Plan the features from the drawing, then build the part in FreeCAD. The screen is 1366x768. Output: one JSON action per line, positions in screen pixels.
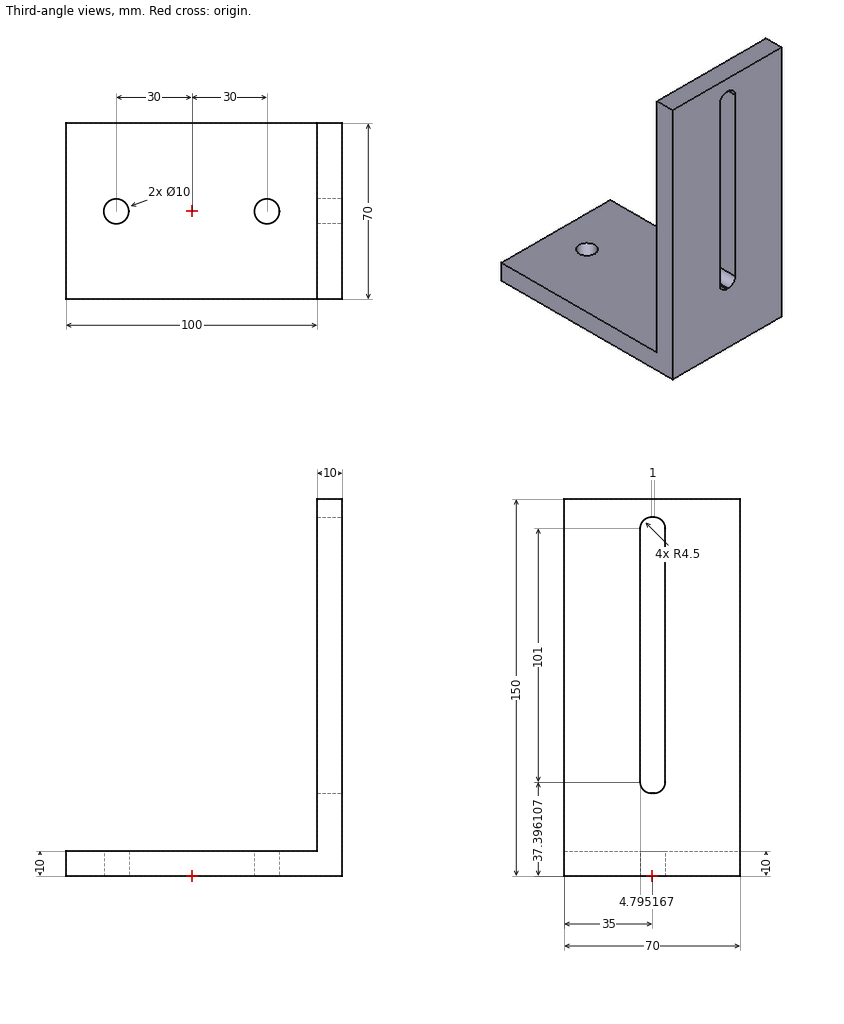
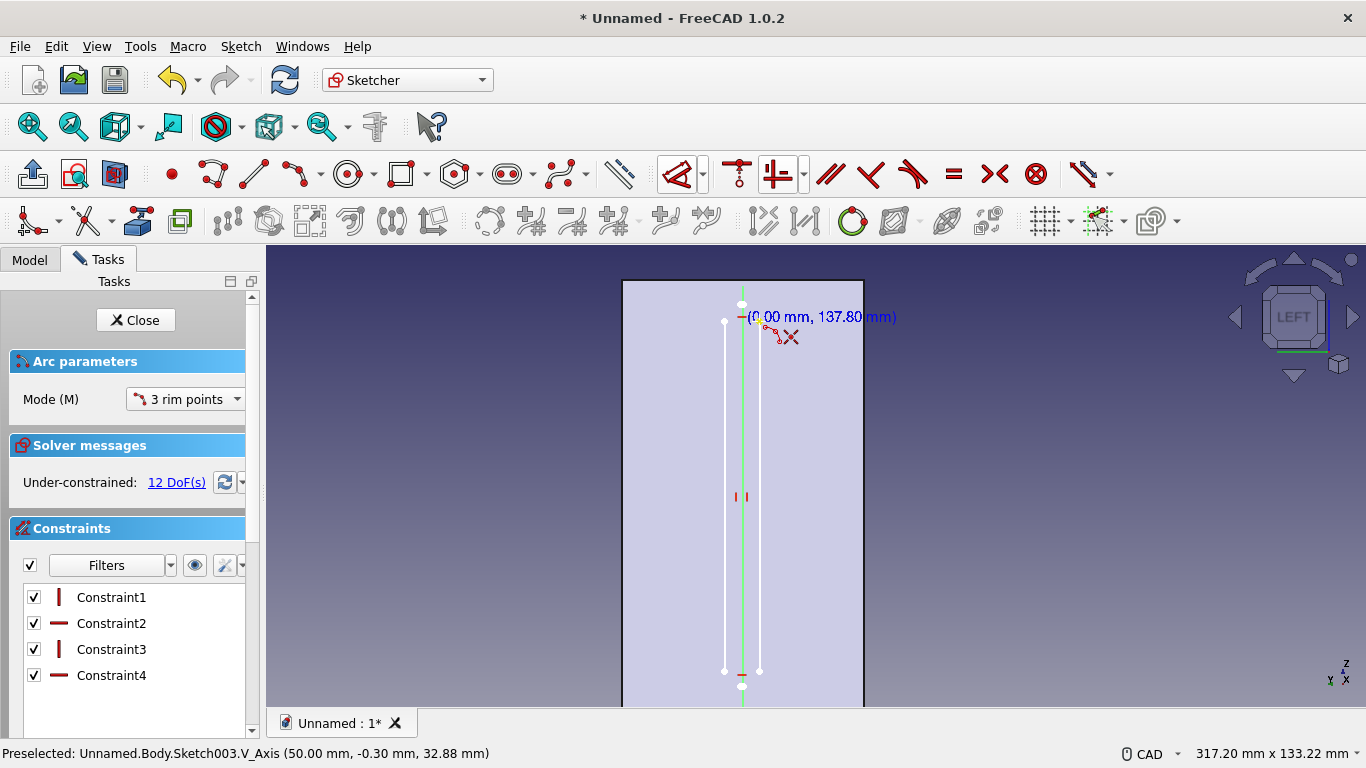
{"action": "left_click", "coordinate": [760, 321]}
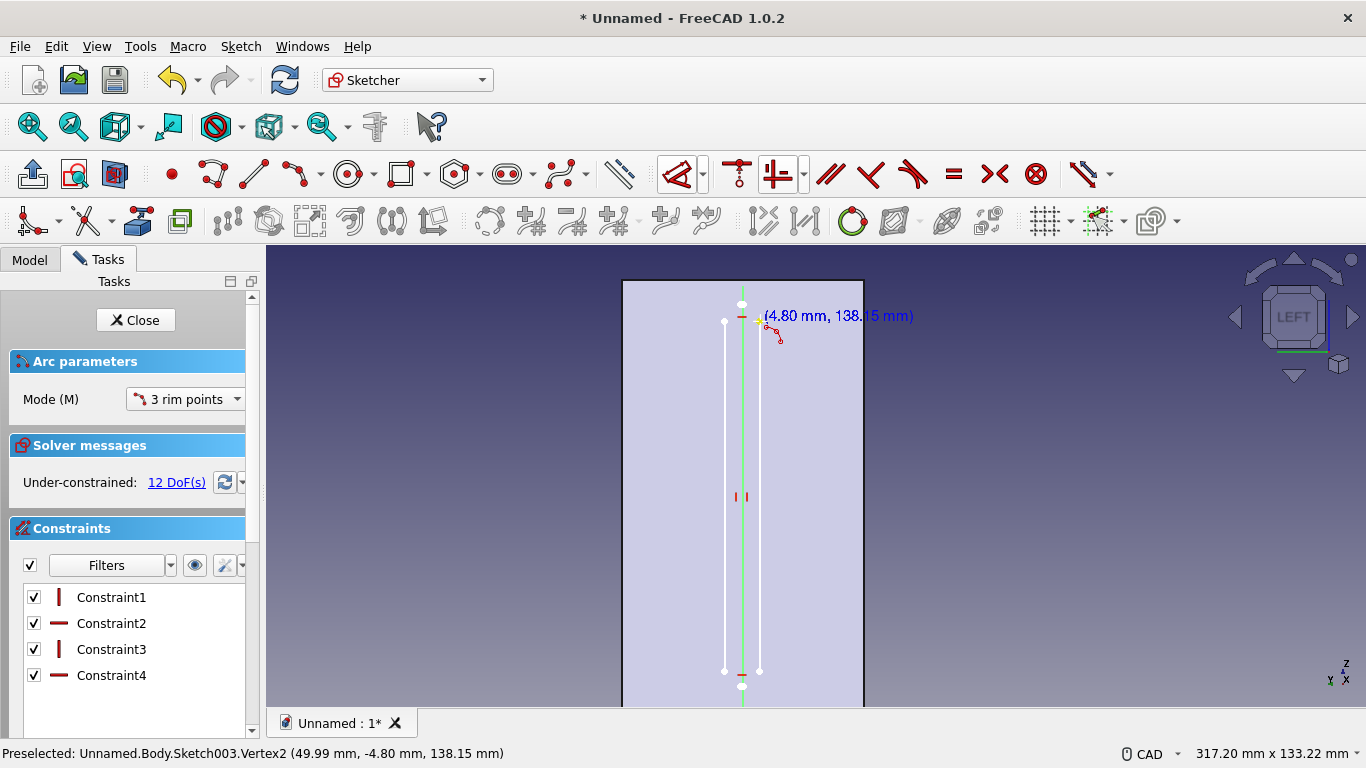
{"action": "scroll", "coordinate": [744, 305], "scroll_direction": "up", "scroll_amount": 14}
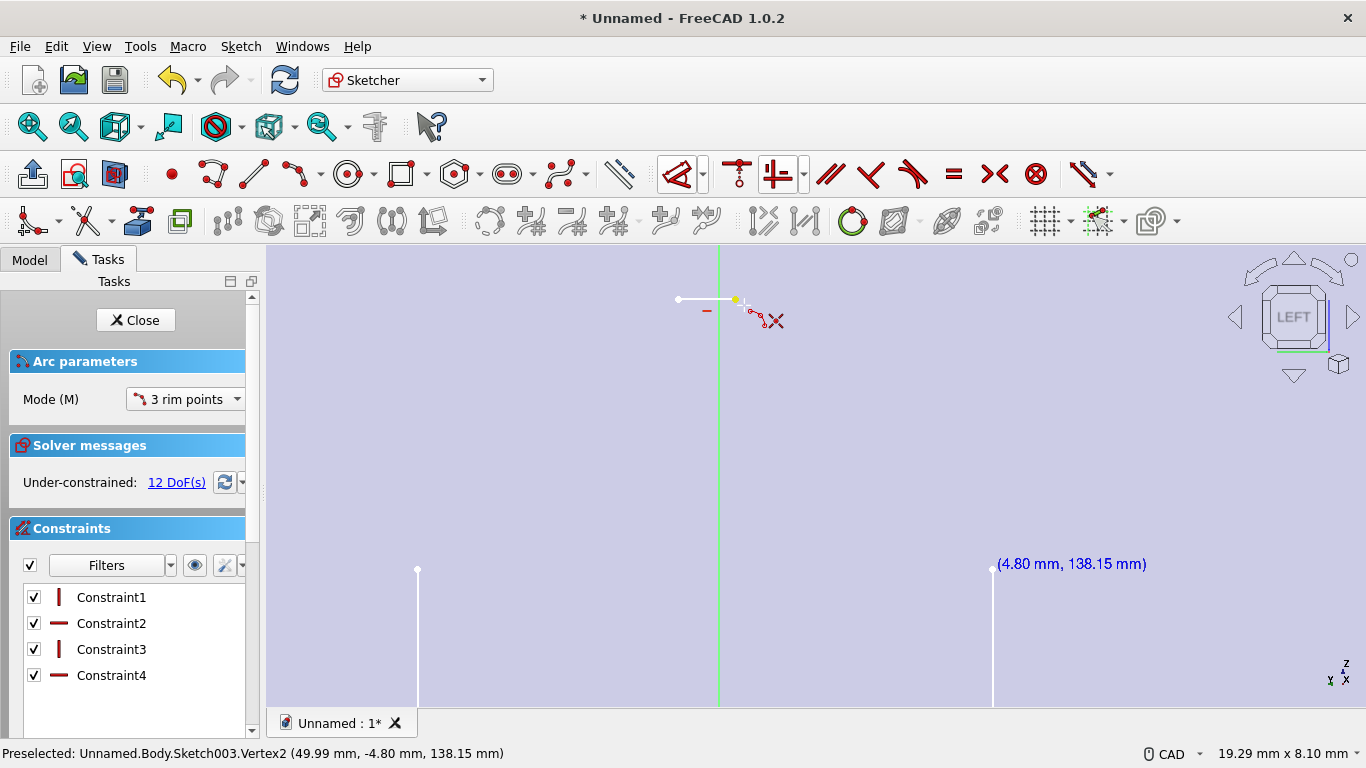
{"action": "left_click", "coordinate": [736, 299]}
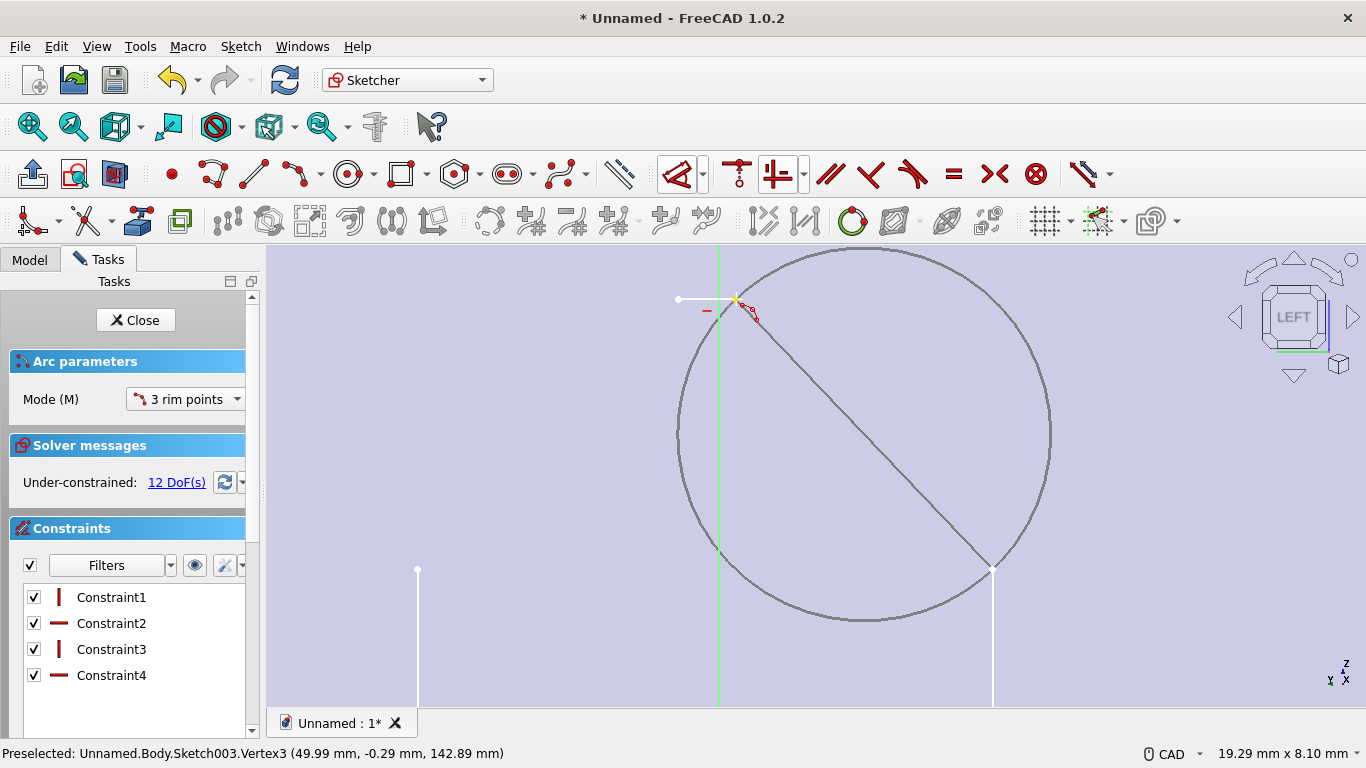
{"action": "scroll", "coordinate": [749, 310], "scroll_direction": "down", "scroll_amount": 16}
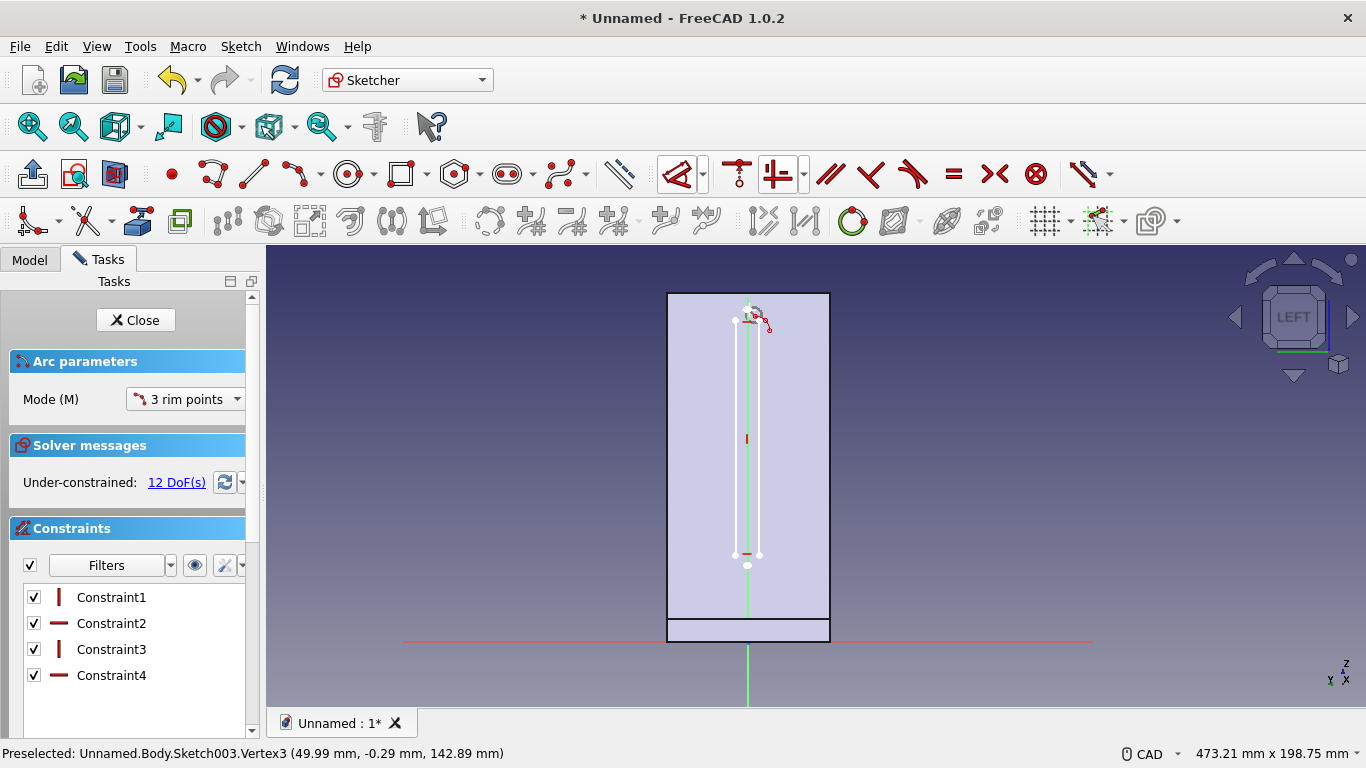
{"action": "scroll", "coordinate": [756, 313], "scroll_direction": "up", "scroll_amount": 9}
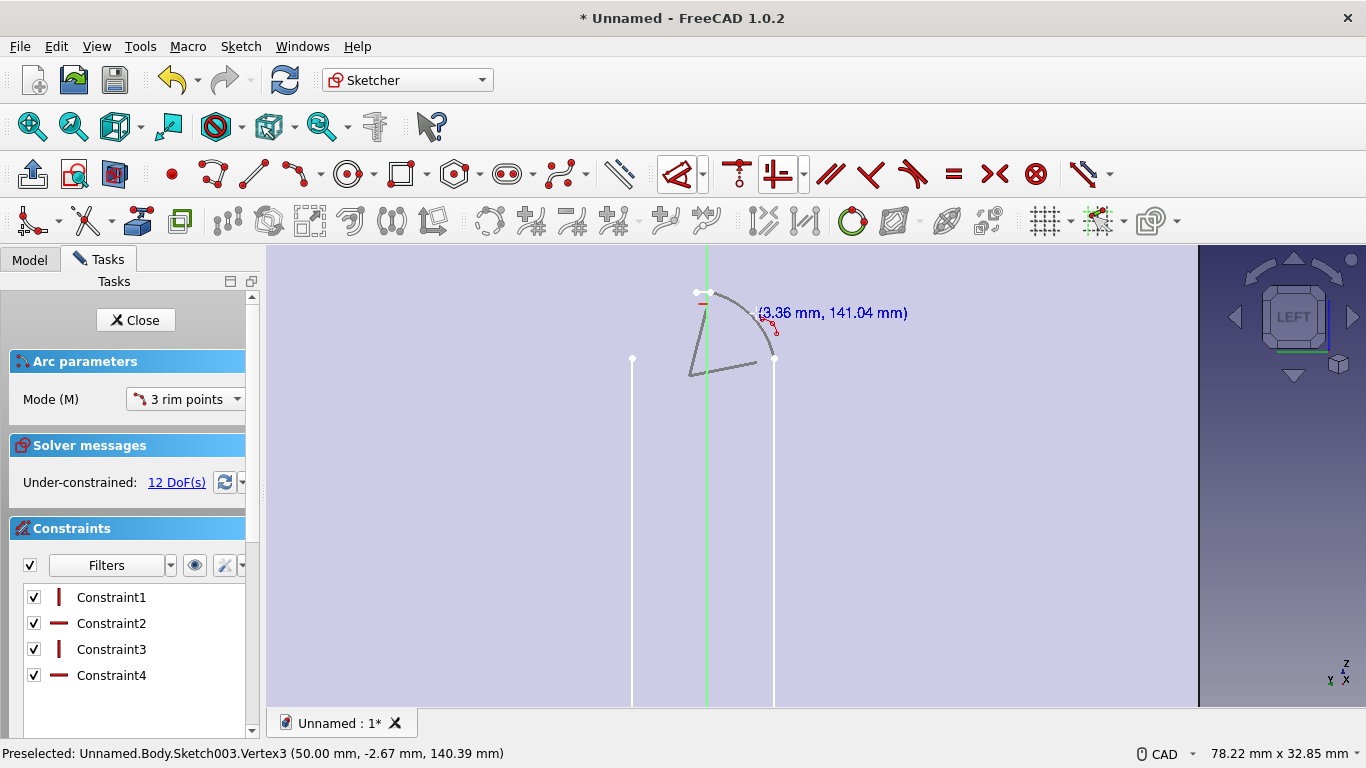
{"action": "left_click", "coordinate": [755, 311]}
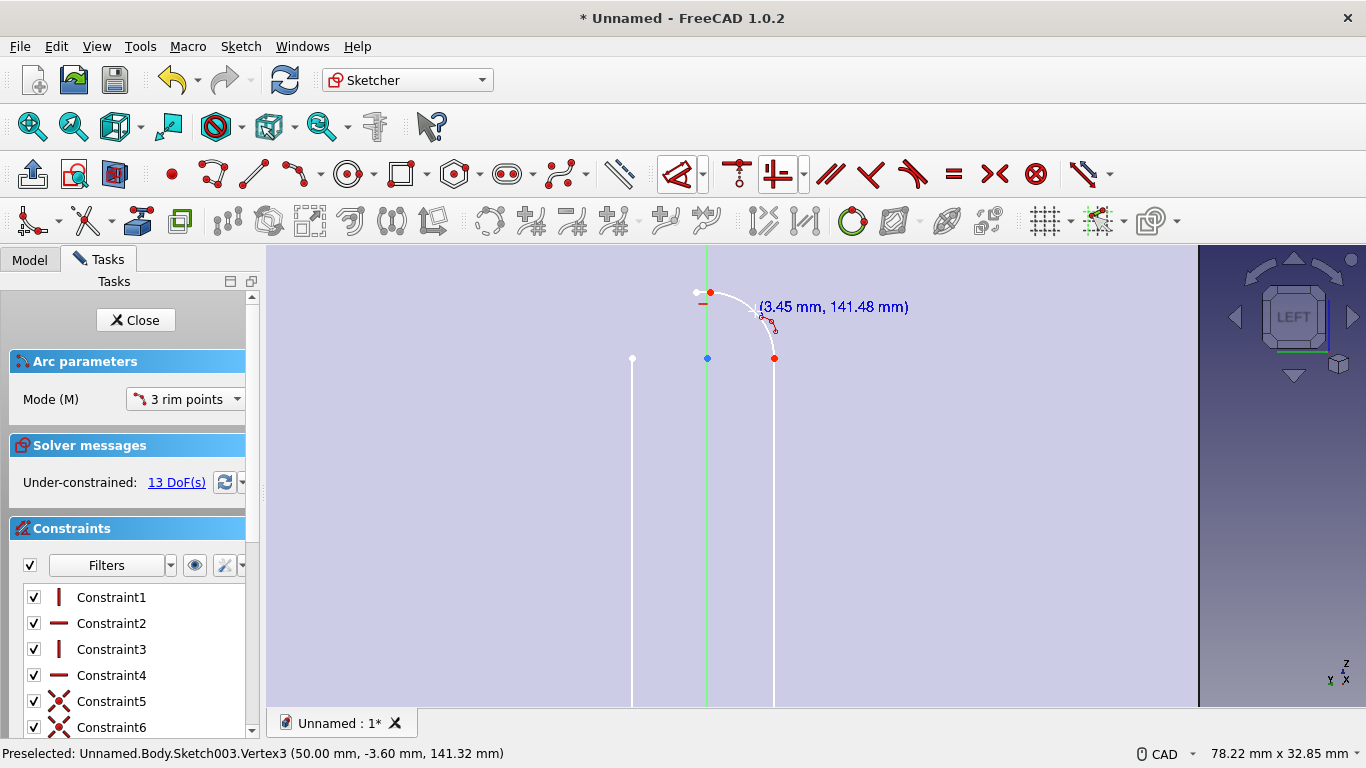
{"action": "scroll", "coordinate": [697, 292], "scroll_direction": "up", "scroll_amount": 5}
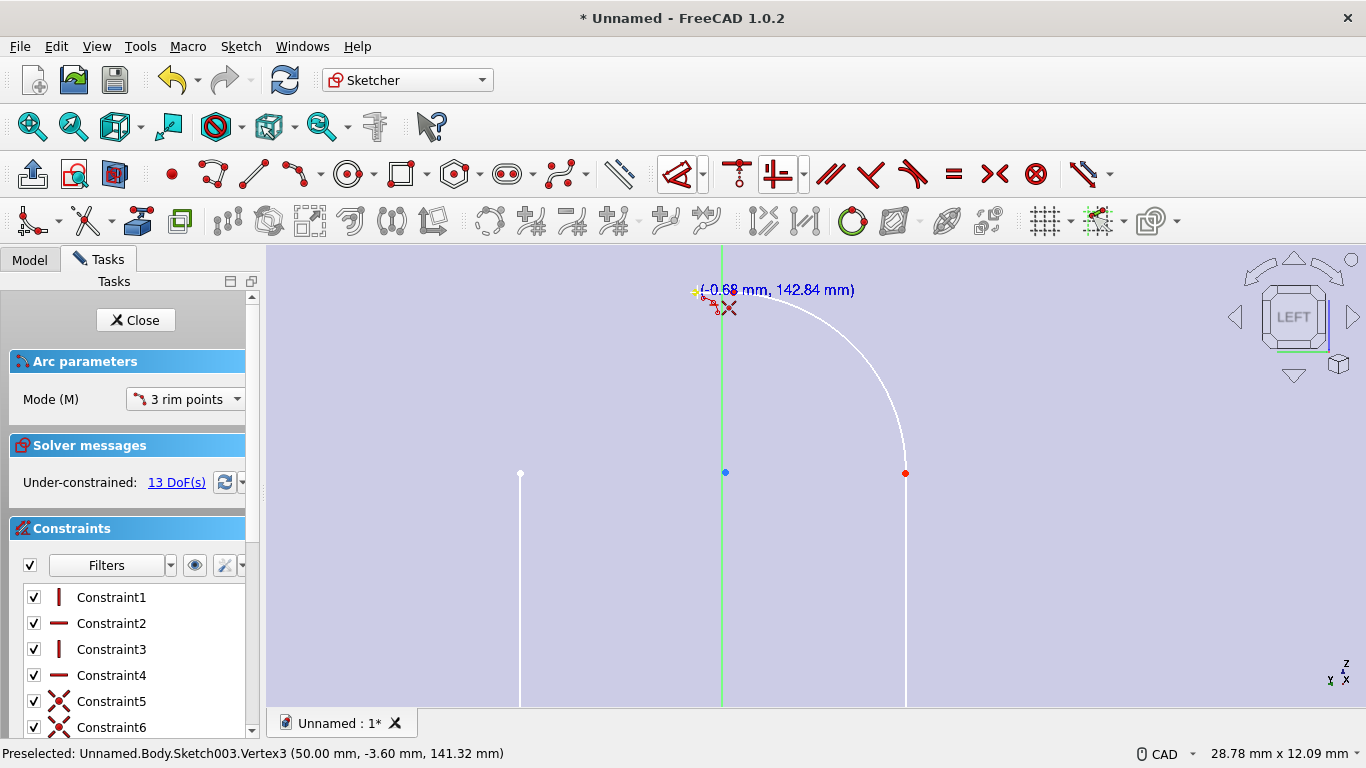
{"action": "left_click", "coordinate": [695, 293]}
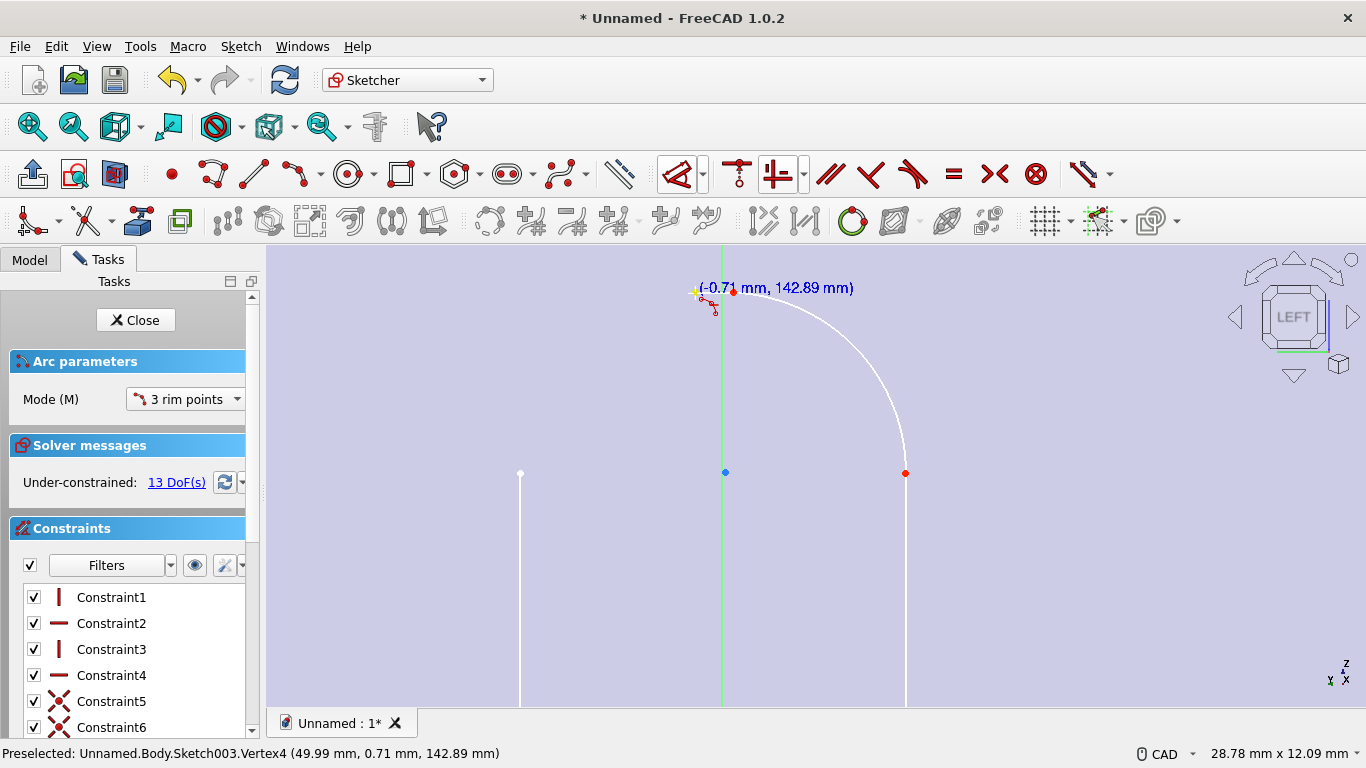
{"action": "scroll", "coordinate": [749, 343], "scroll_direction": "down", "scroll_amount": 15}